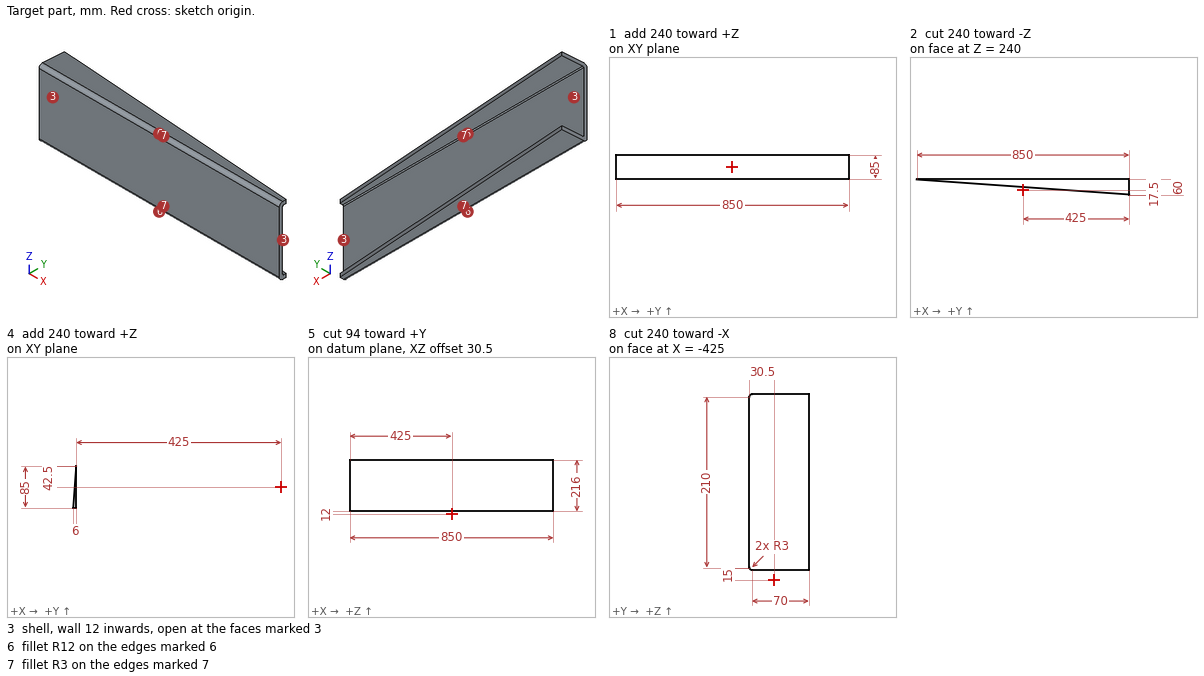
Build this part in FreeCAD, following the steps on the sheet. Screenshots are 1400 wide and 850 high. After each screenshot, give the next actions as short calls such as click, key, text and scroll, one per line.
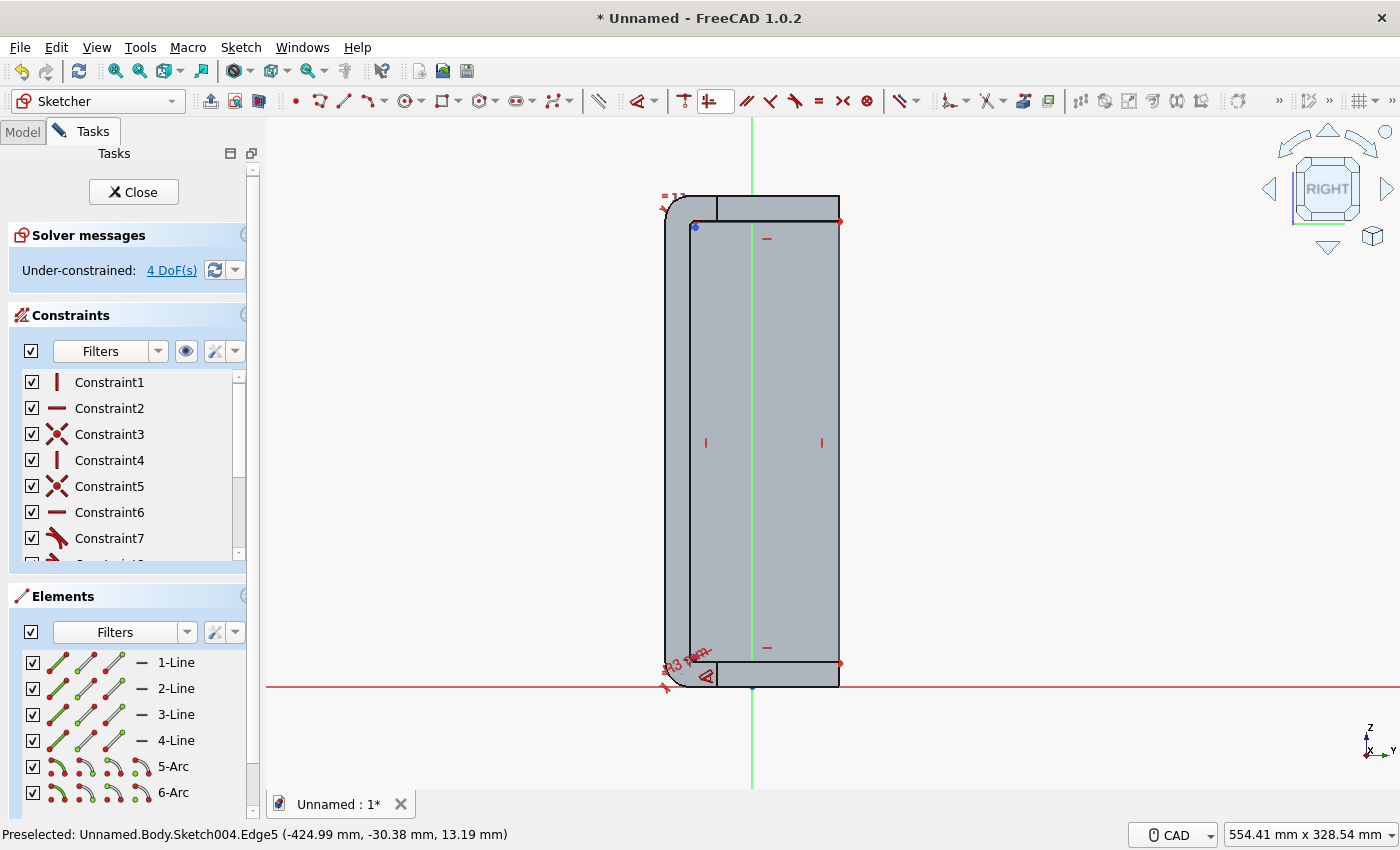
click(739, 664)
click(767, 630)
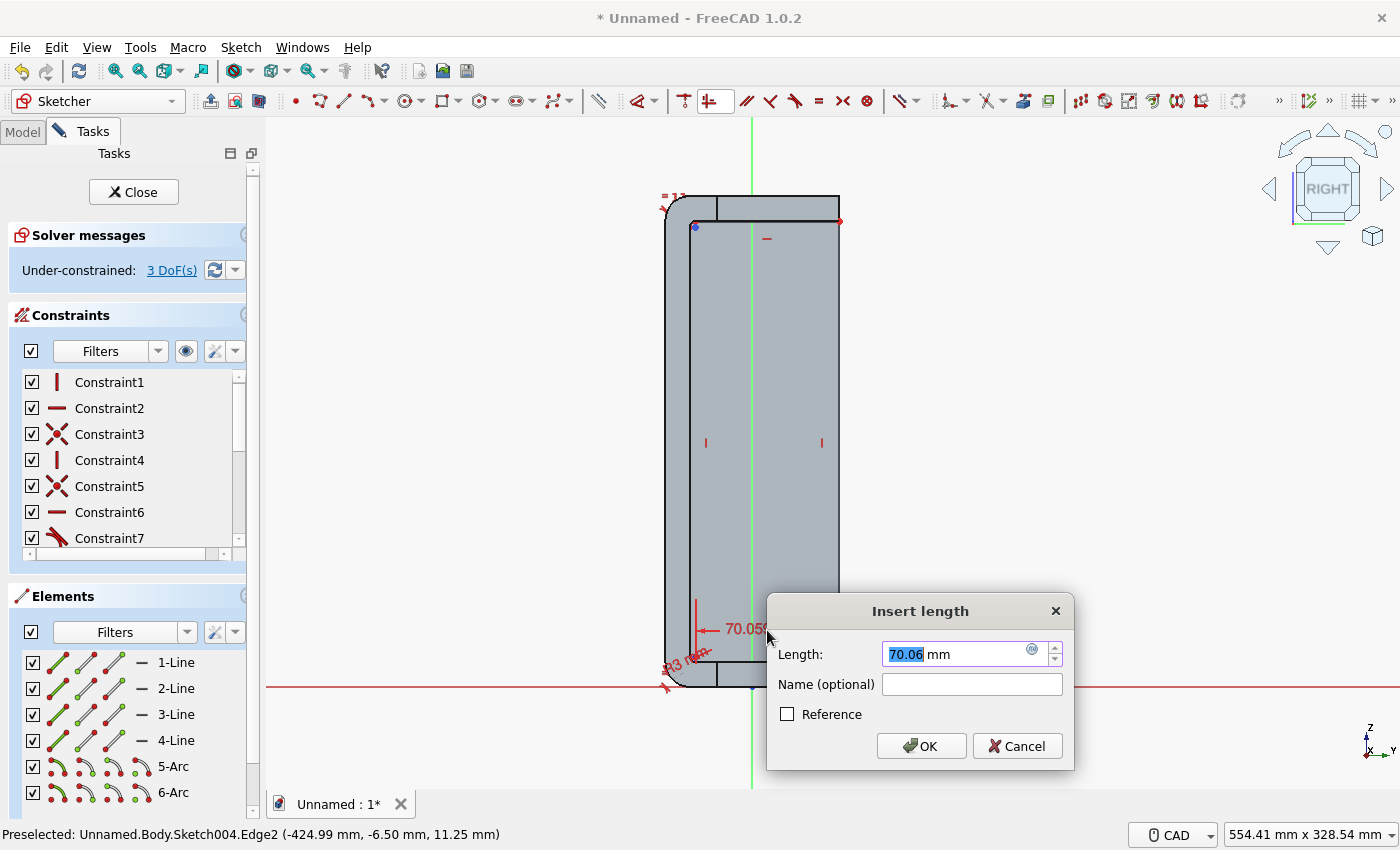
text(70)
key(Return)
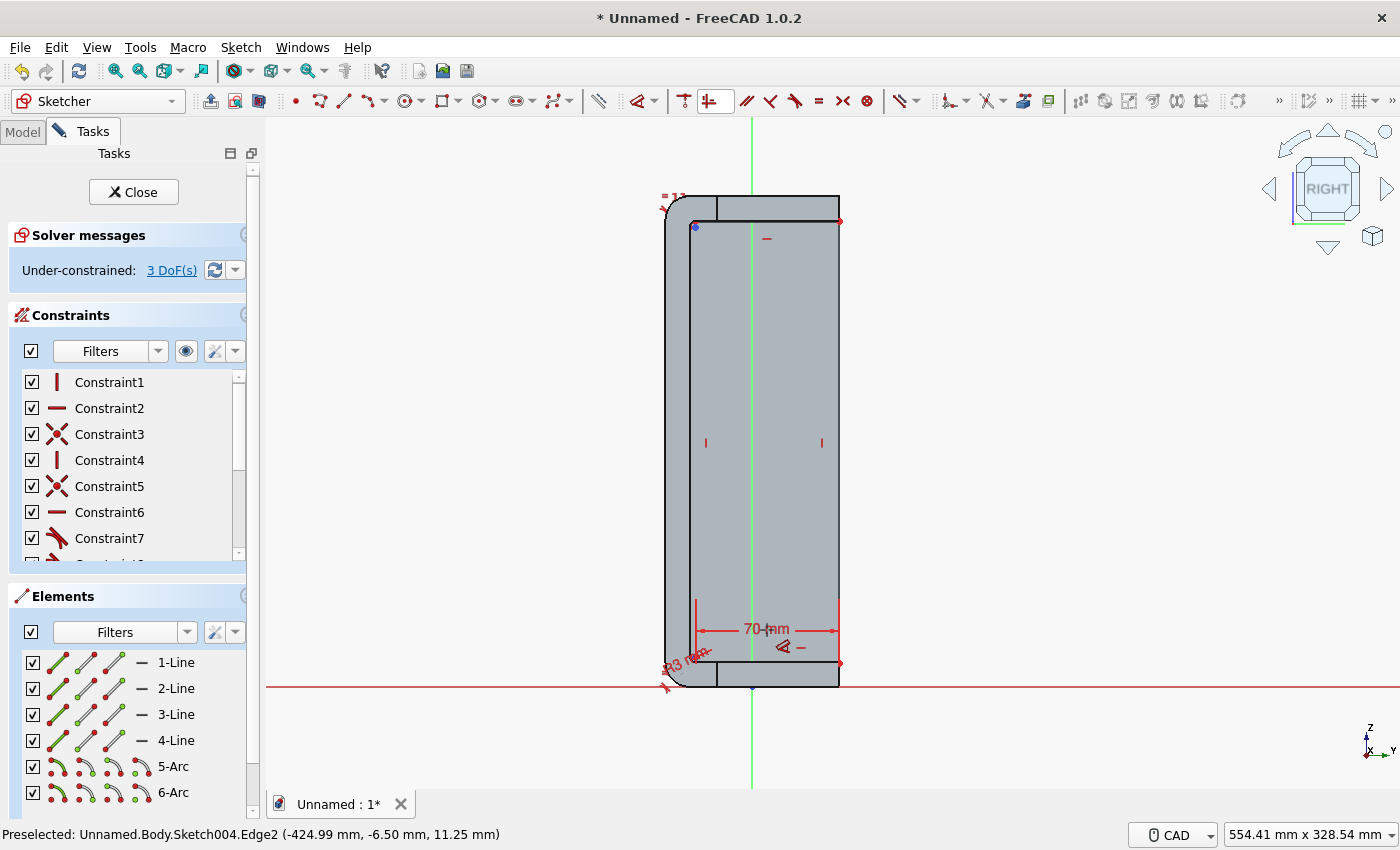
click(690, 357)
click(656, 443)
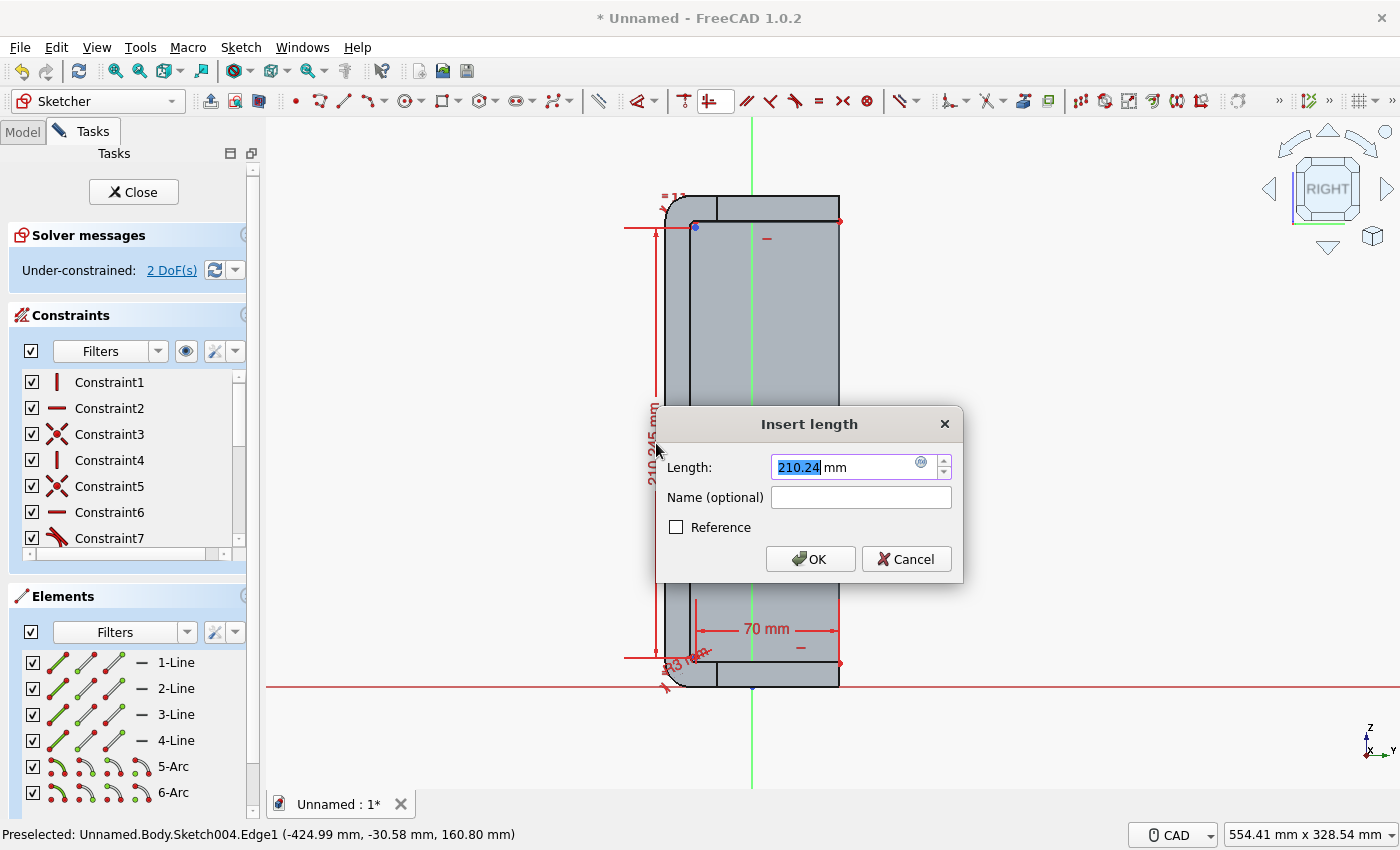
text(210)
key(Return)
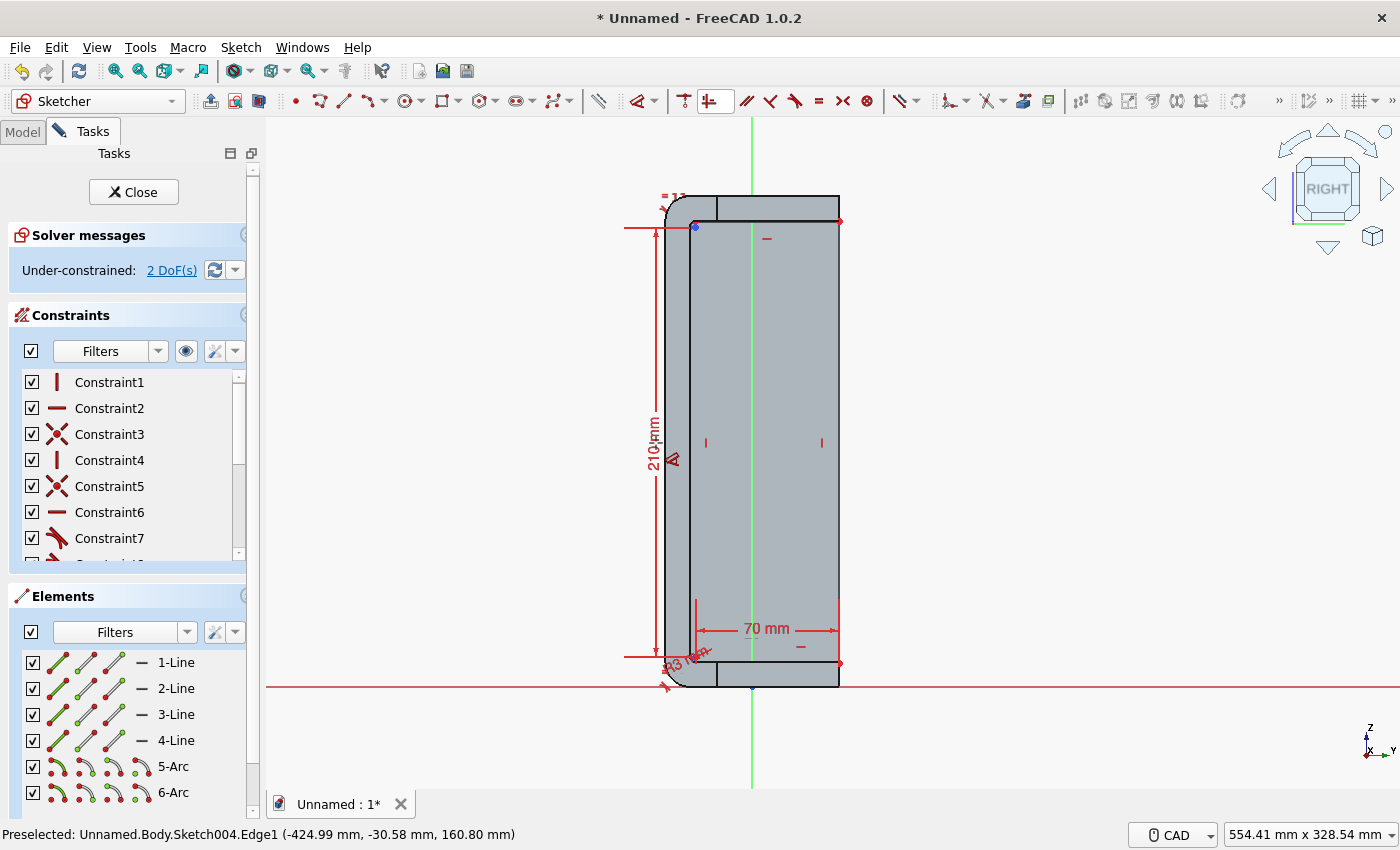
scroll(690, 657, up, 4)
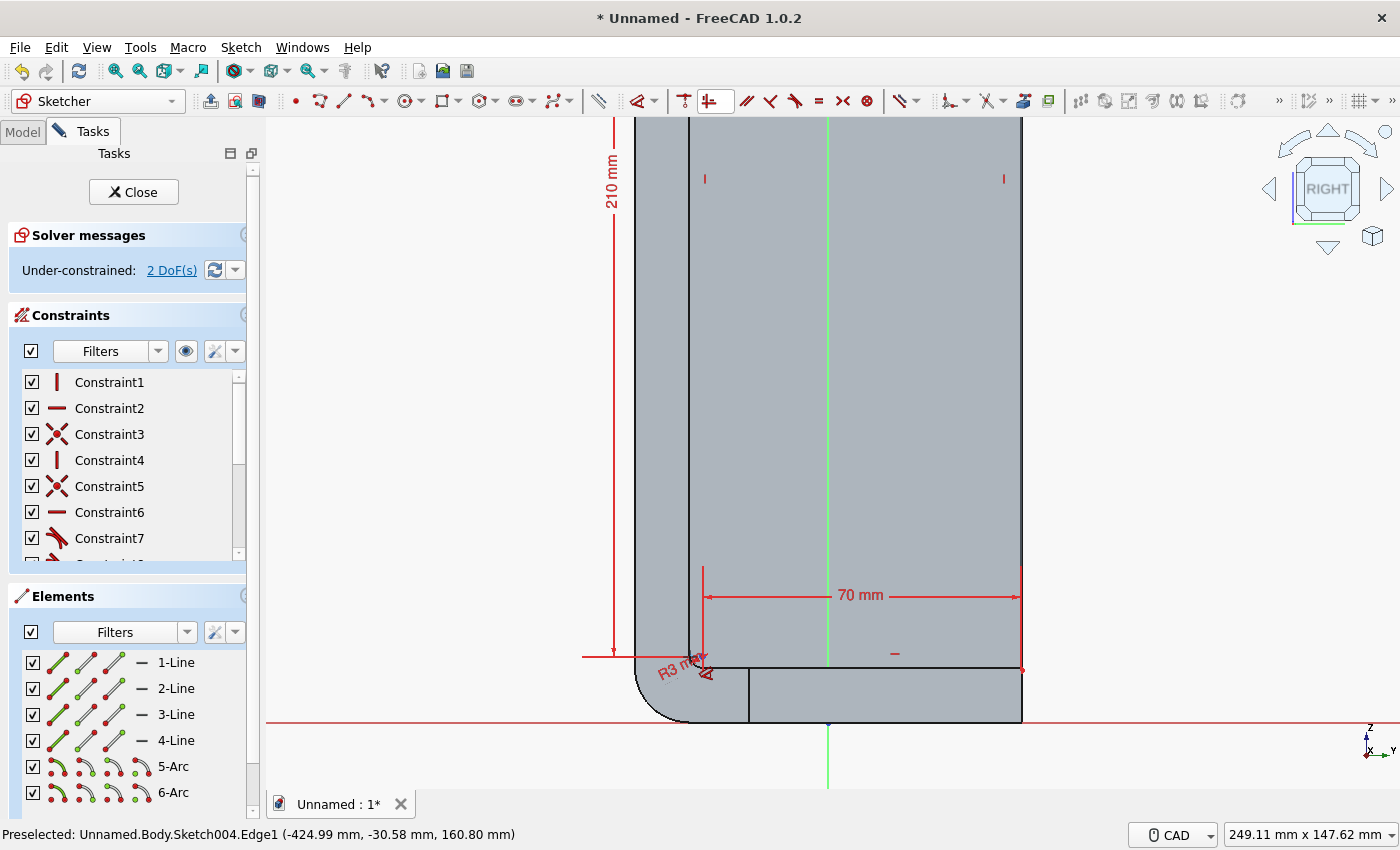
click(689, 657)
click(655, 690)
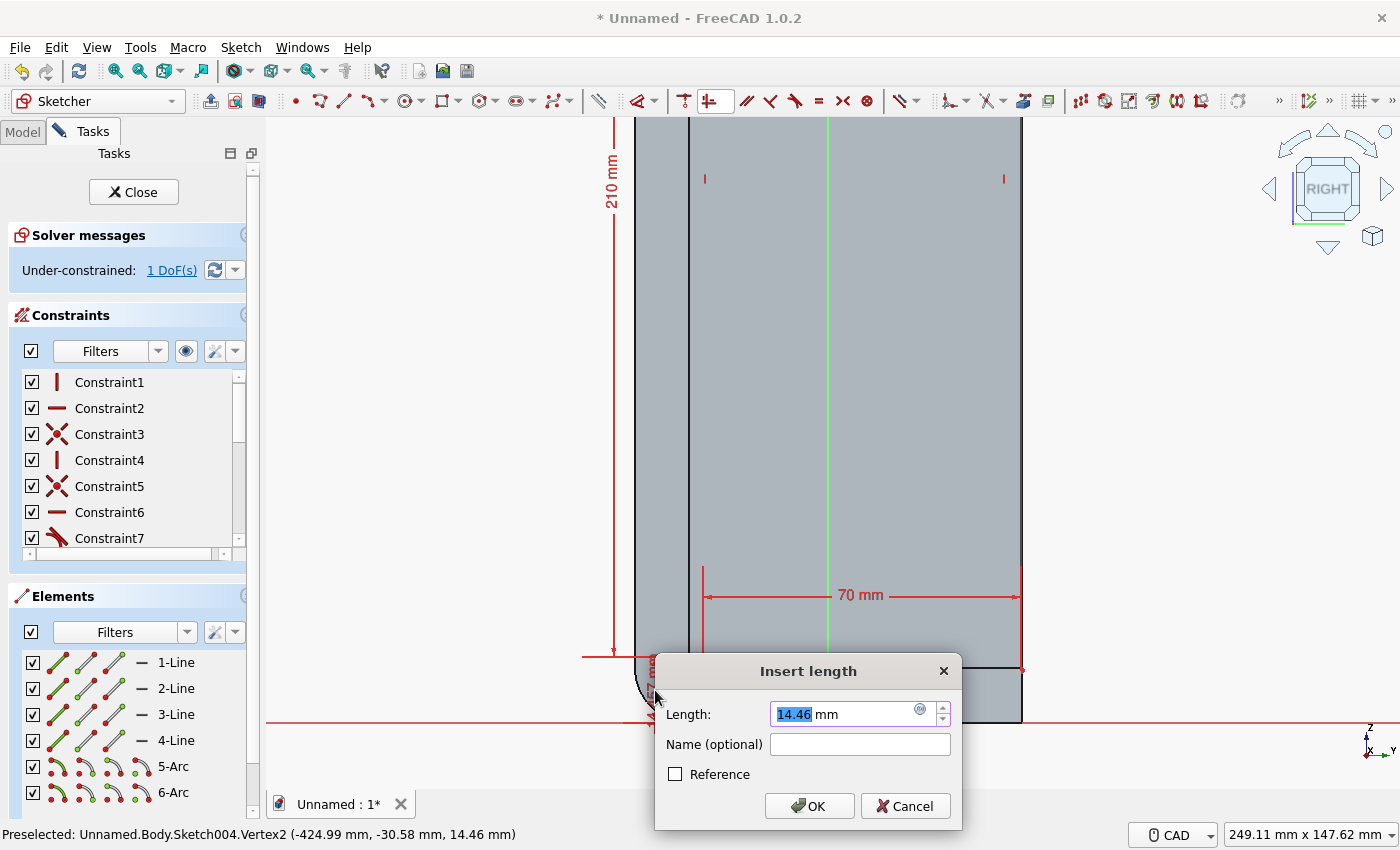
text(15)
key(Return)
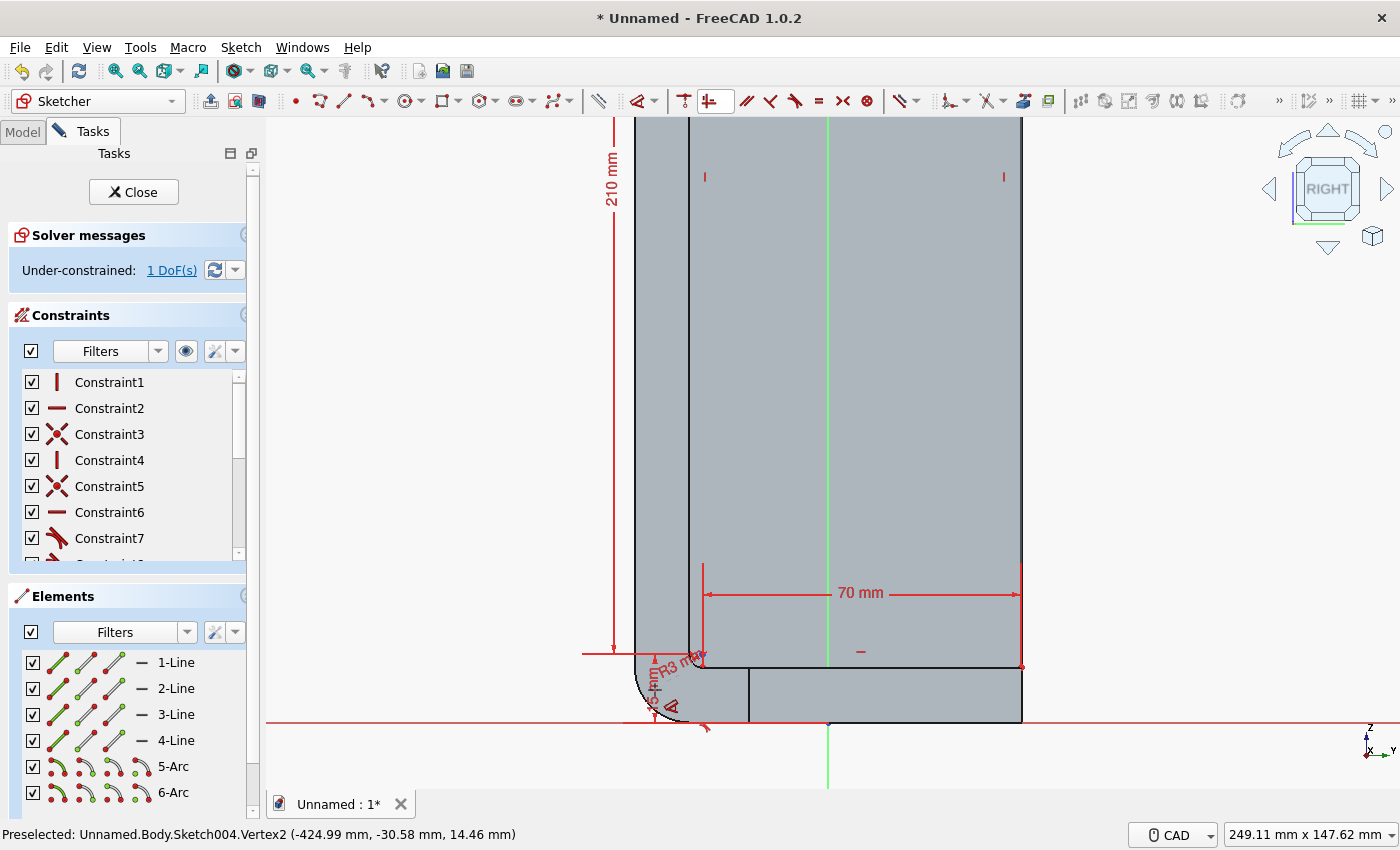
scroll(690, 656, down, 4)